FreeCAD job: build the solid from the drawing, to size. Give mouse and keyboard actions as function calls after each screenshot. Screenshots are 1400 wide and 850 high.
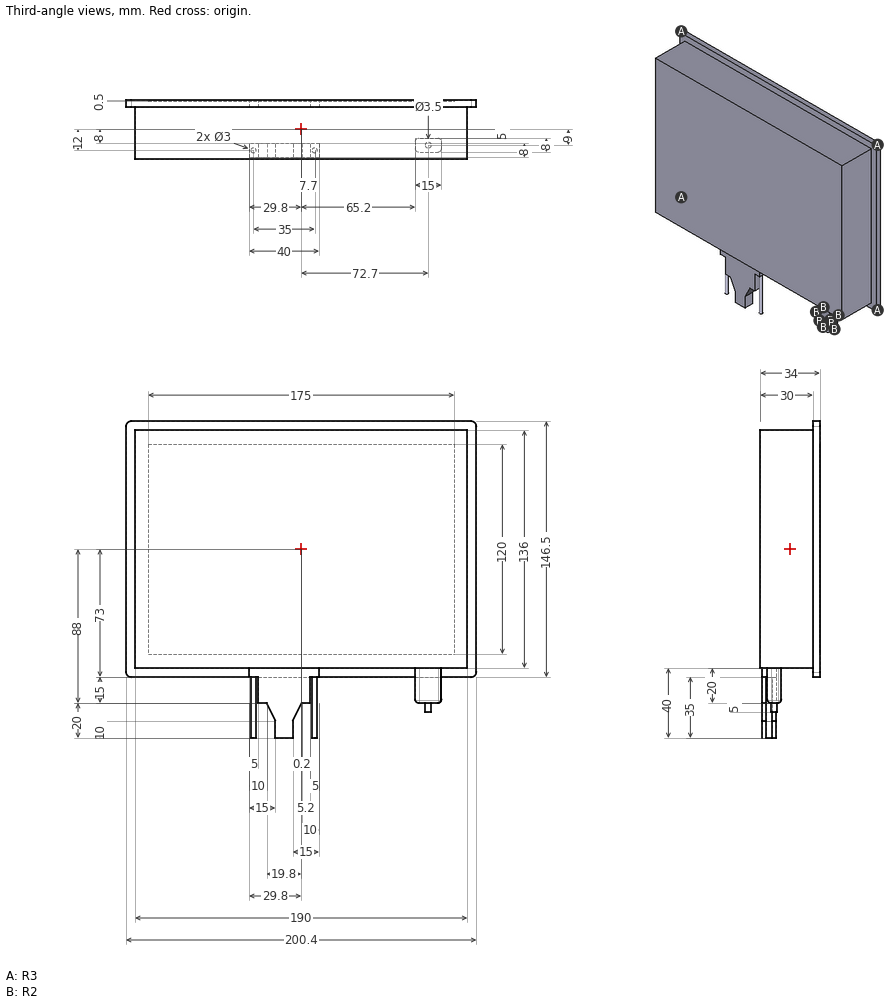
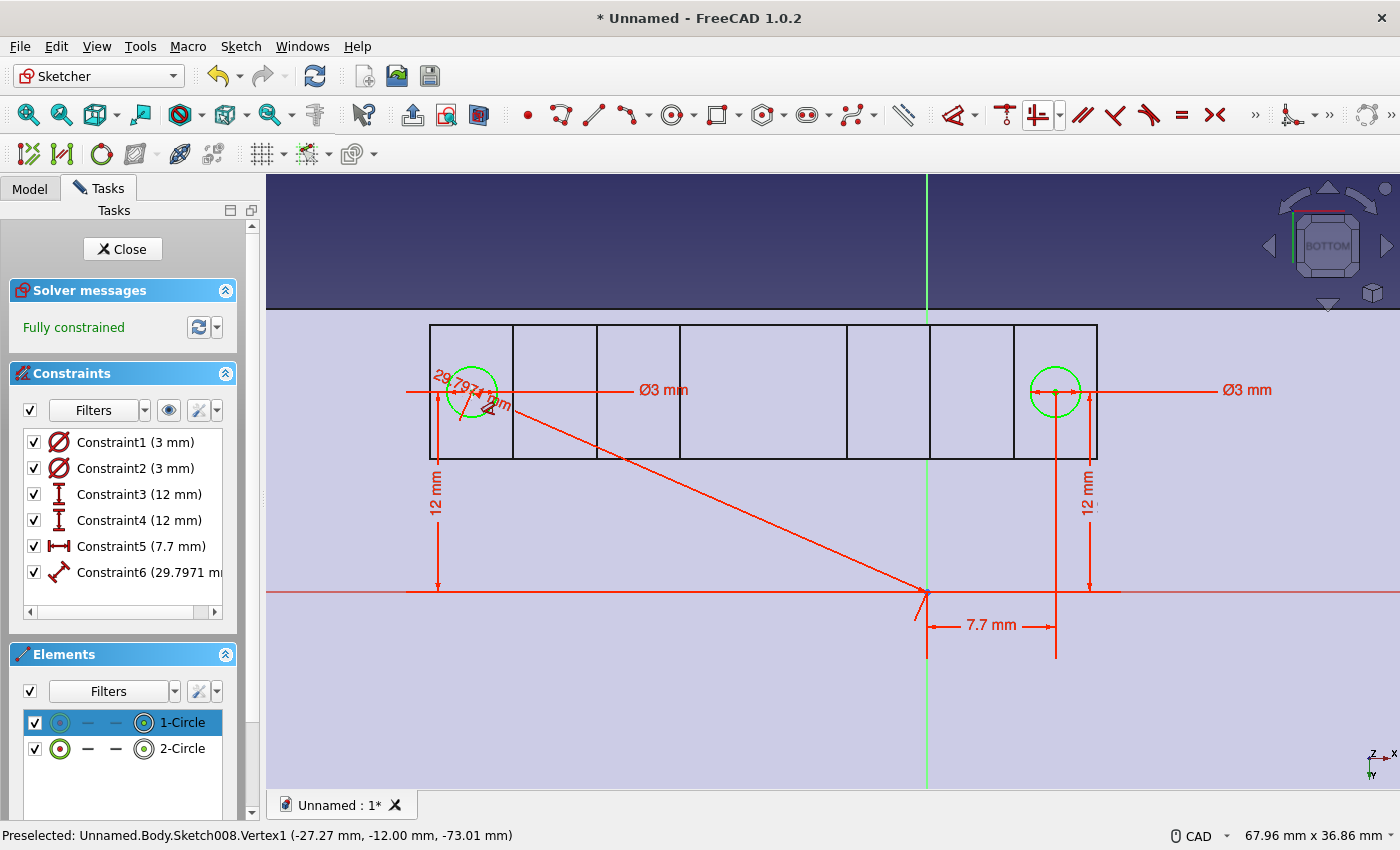
click(1056, 392)
click(764, 358)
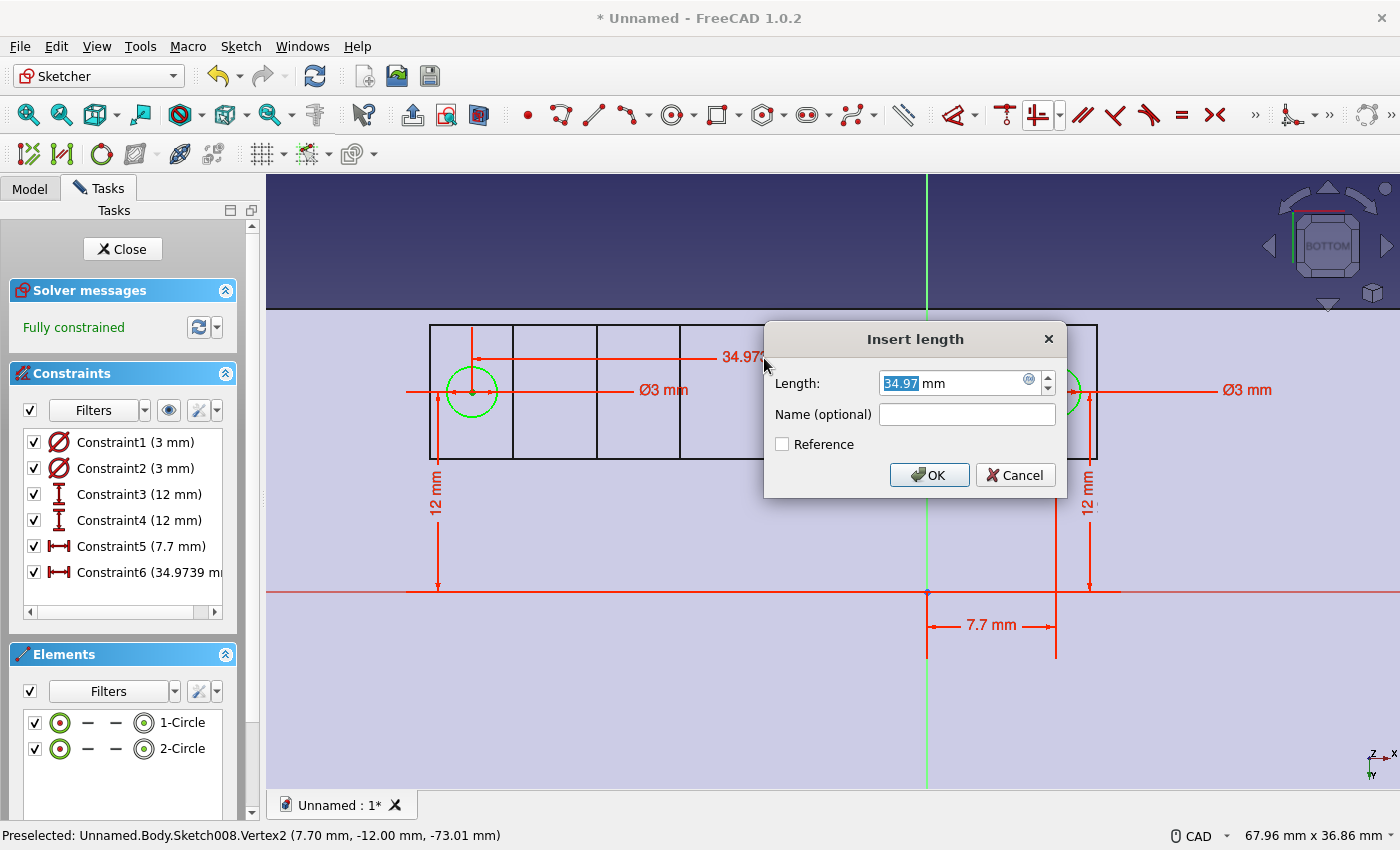
text(35)
key(Return)
key(Escape)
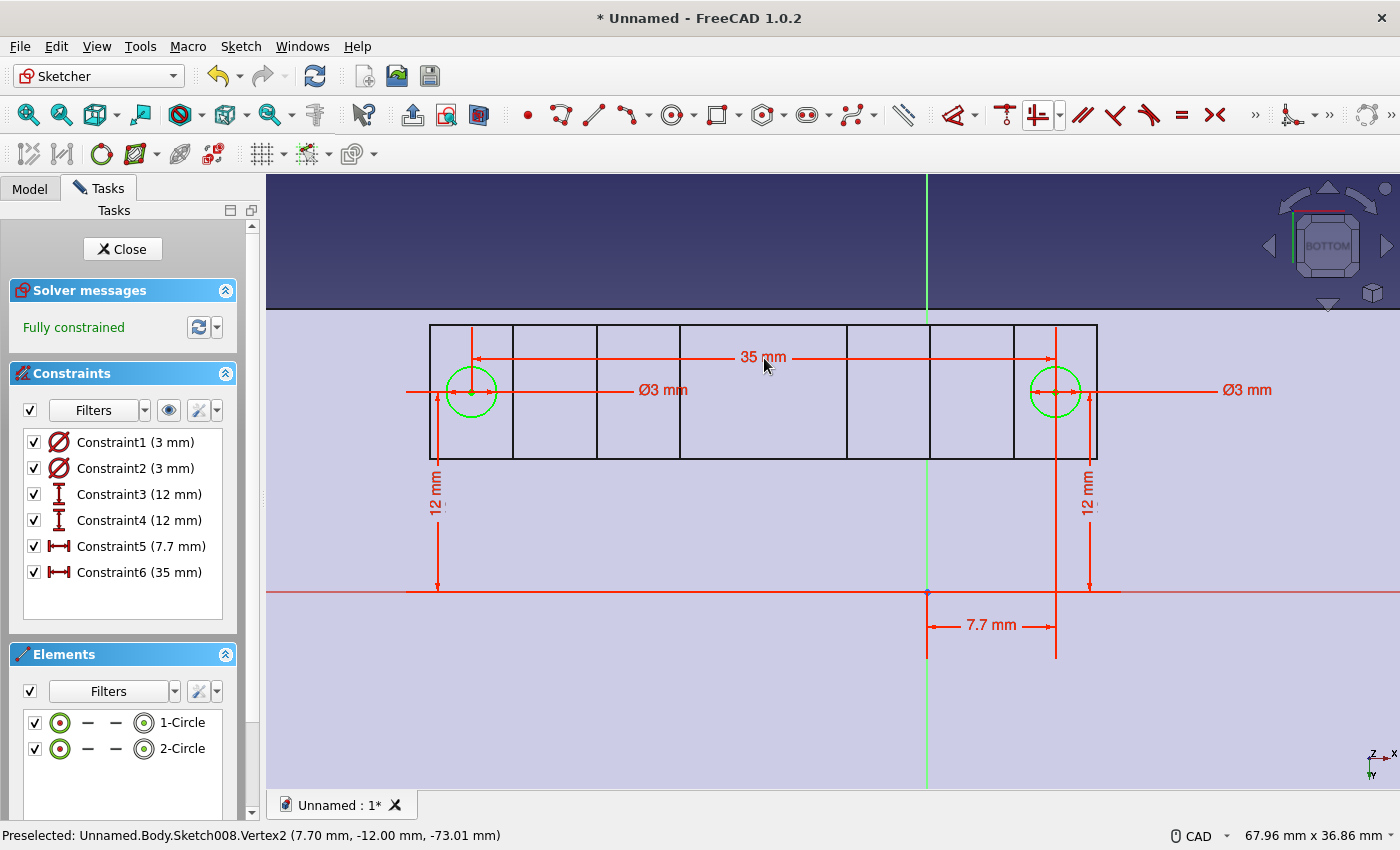
click(123, 249)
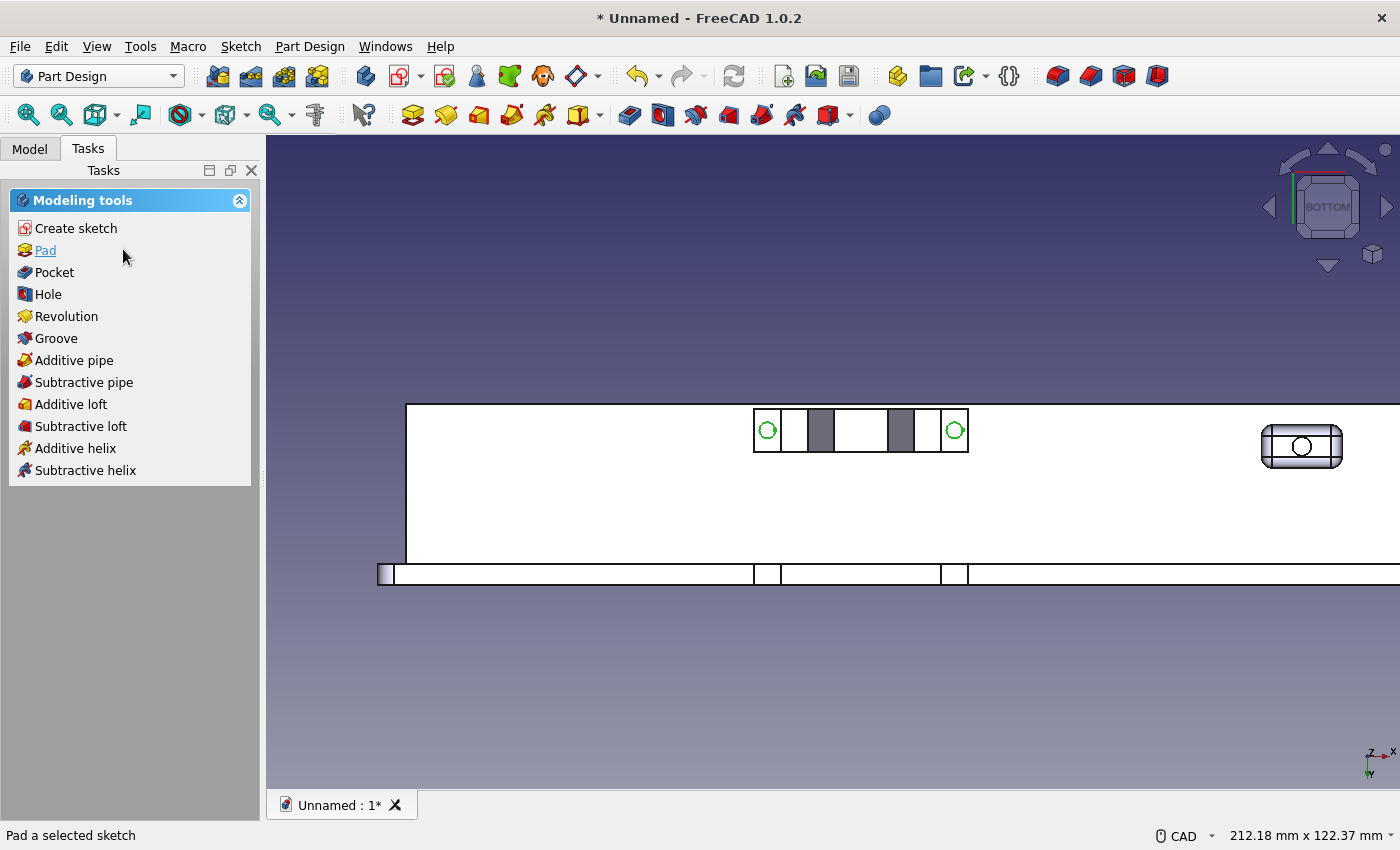
click(413, 116)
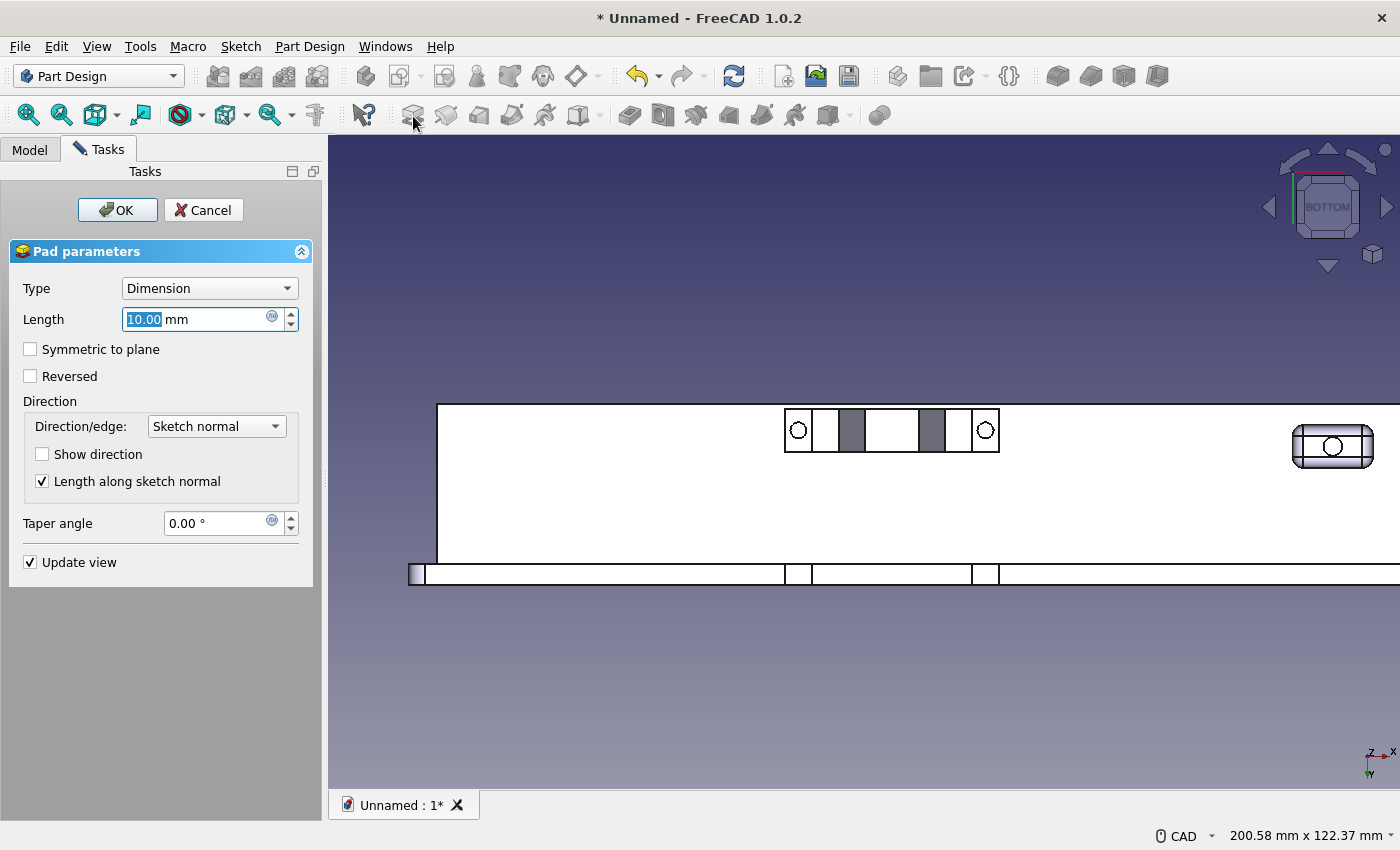
text(35)
key(Tab)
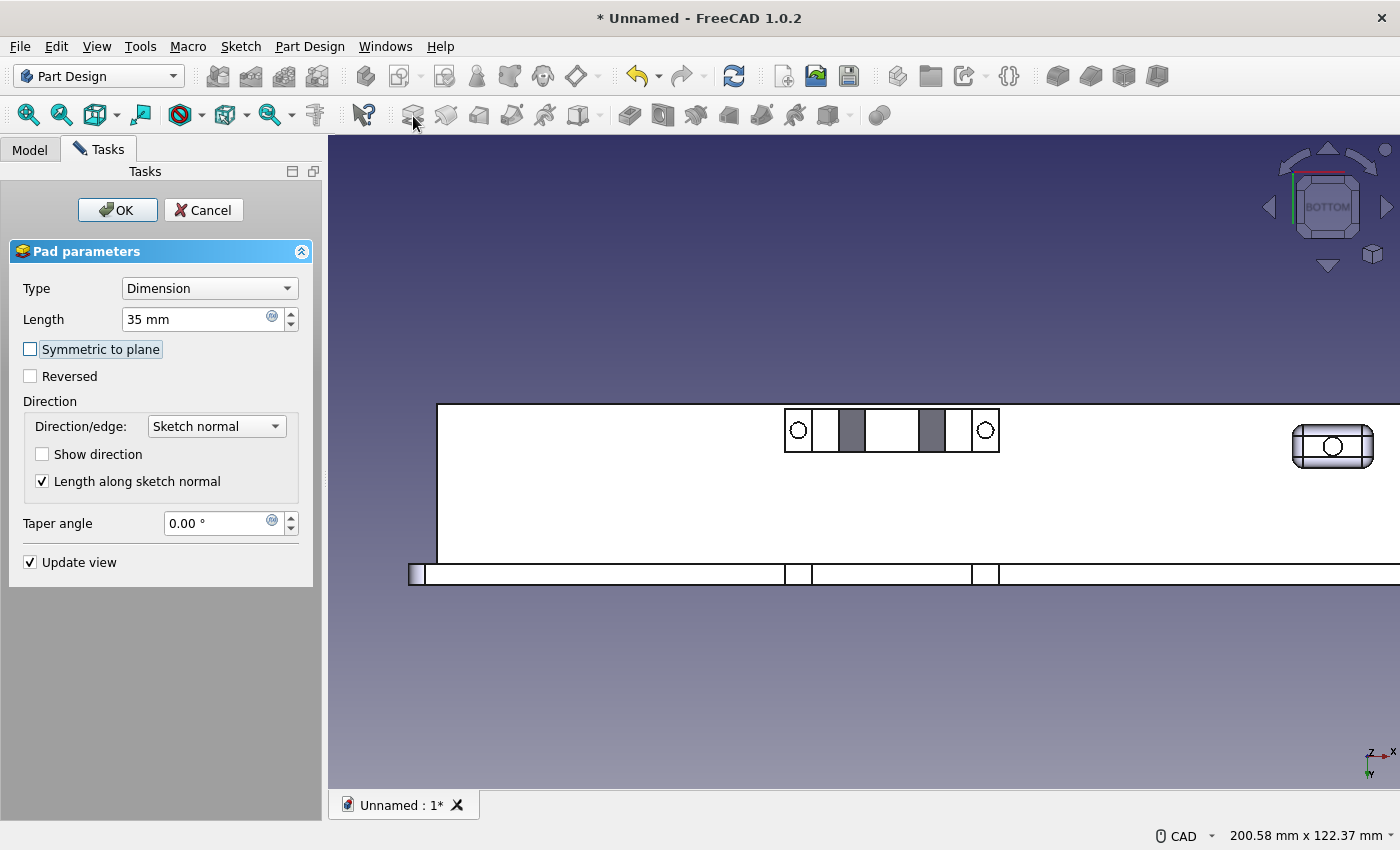
click(118, 210)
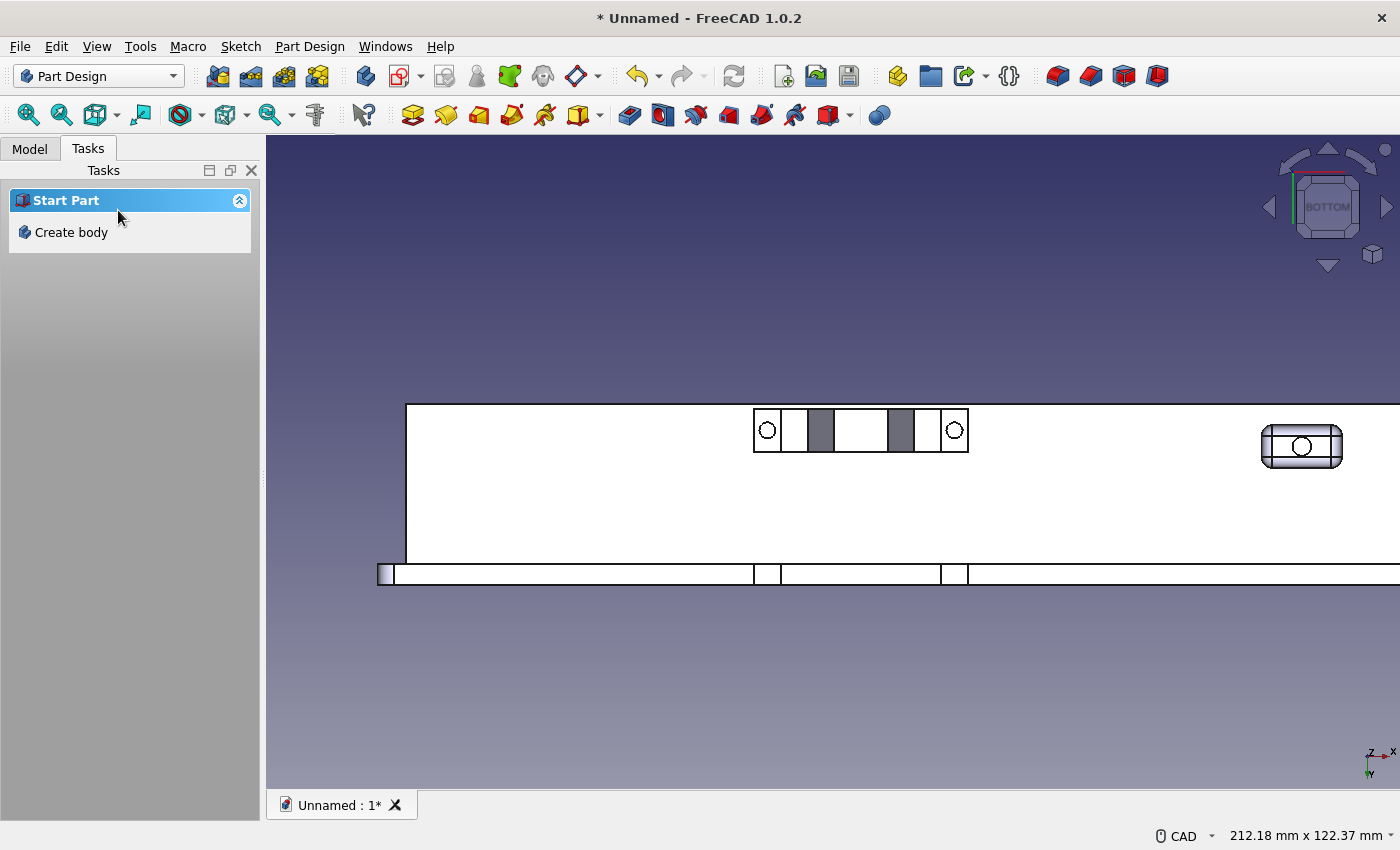
key(0)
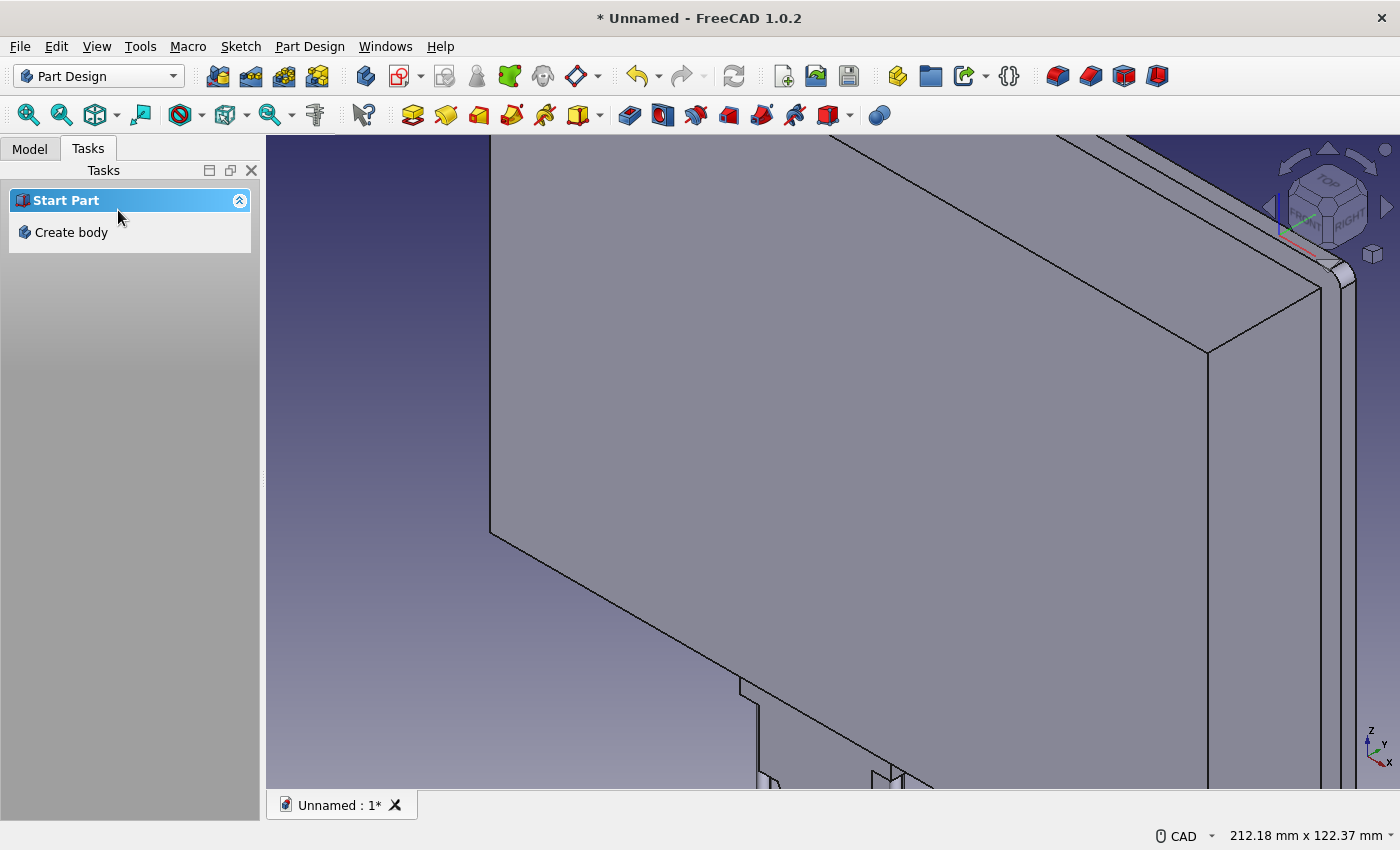
click(29, 116)